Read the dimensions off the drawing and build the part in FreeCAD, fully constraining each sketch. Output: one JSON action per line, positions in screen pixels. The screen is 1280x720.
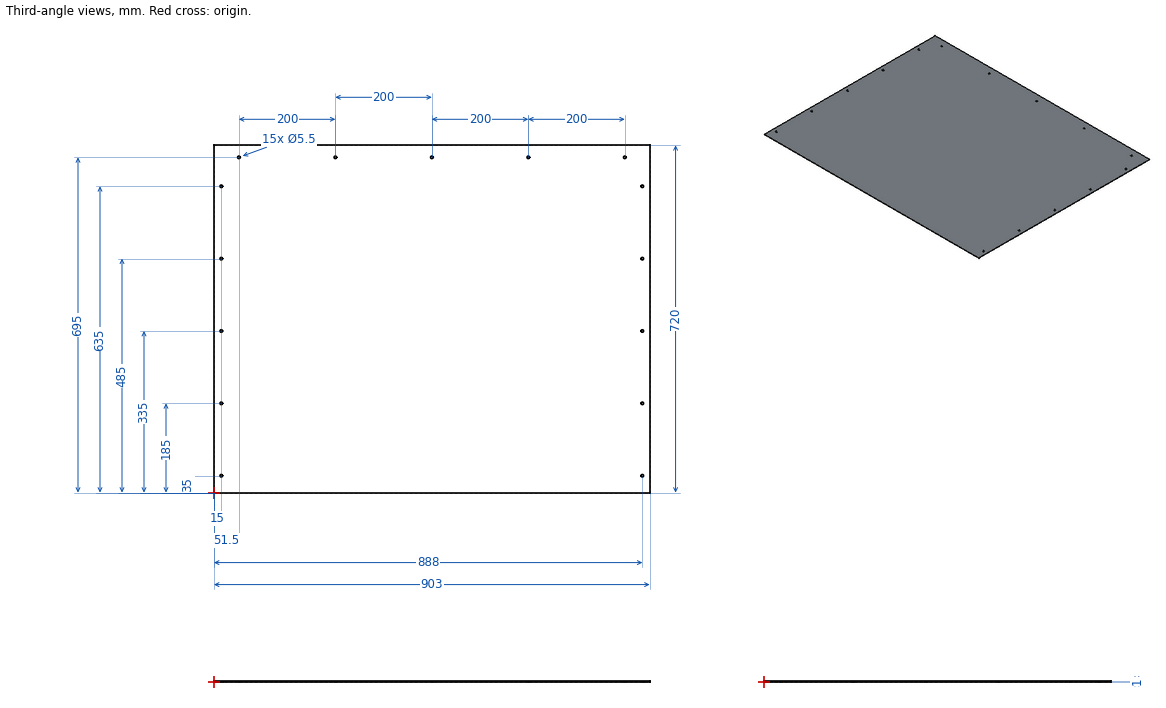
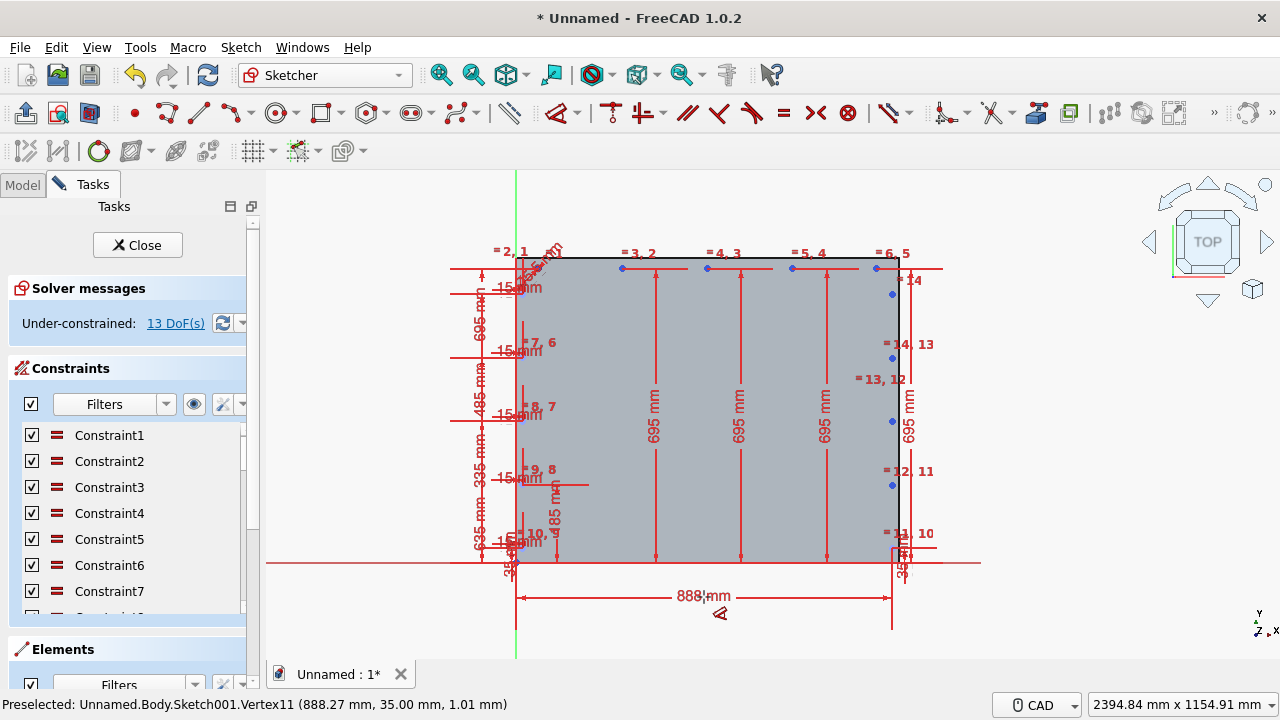
{"action": "left_click", "coordinate": [892, 486]}
{"action": "left_click", "coordinate": [618, 597]}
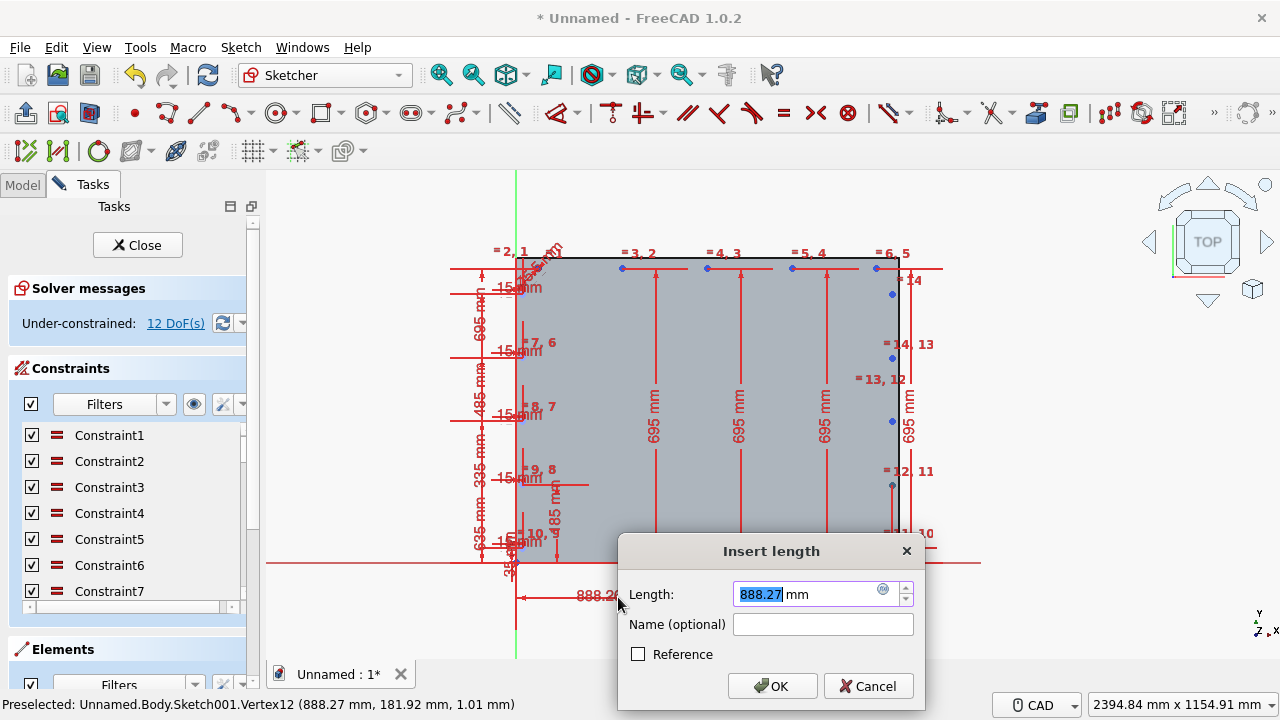
{"action": "type", "text": "888"}
{"action": "key", "text": "Return"}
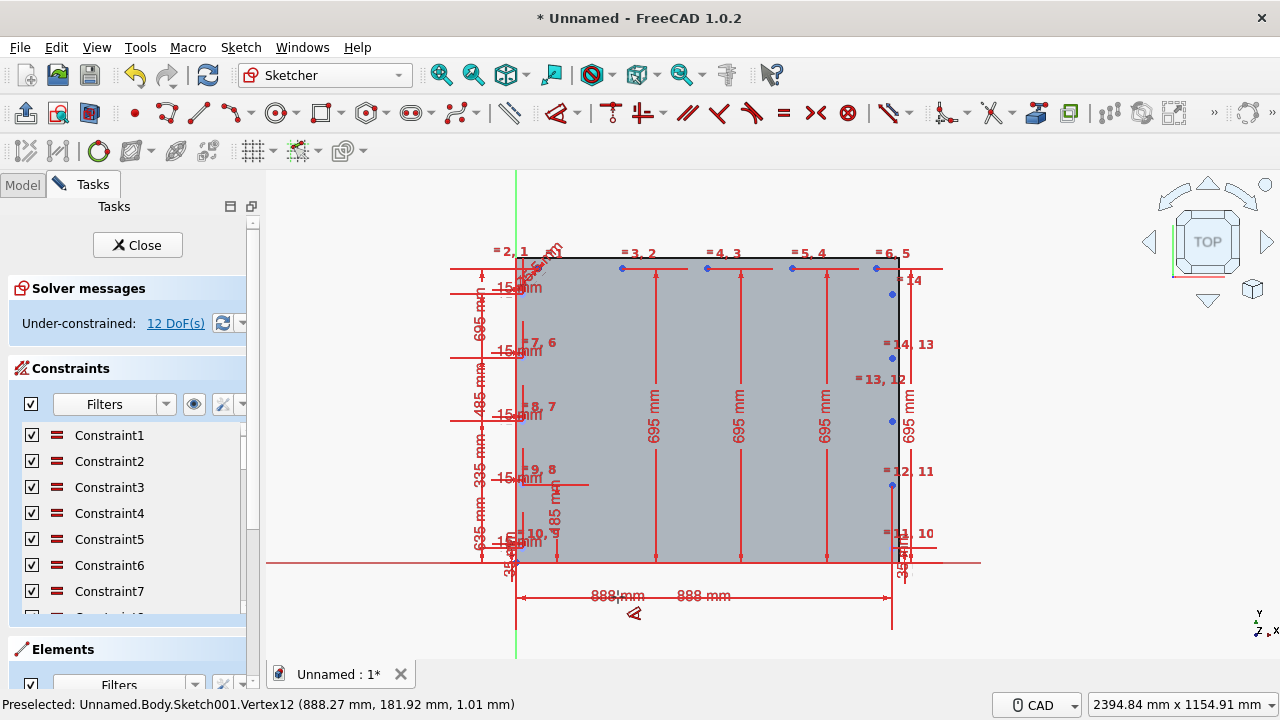
{"action": "left_click", "coordinate": [892, 486]}
{"action": "left_click", "coordinate": [926, 524]}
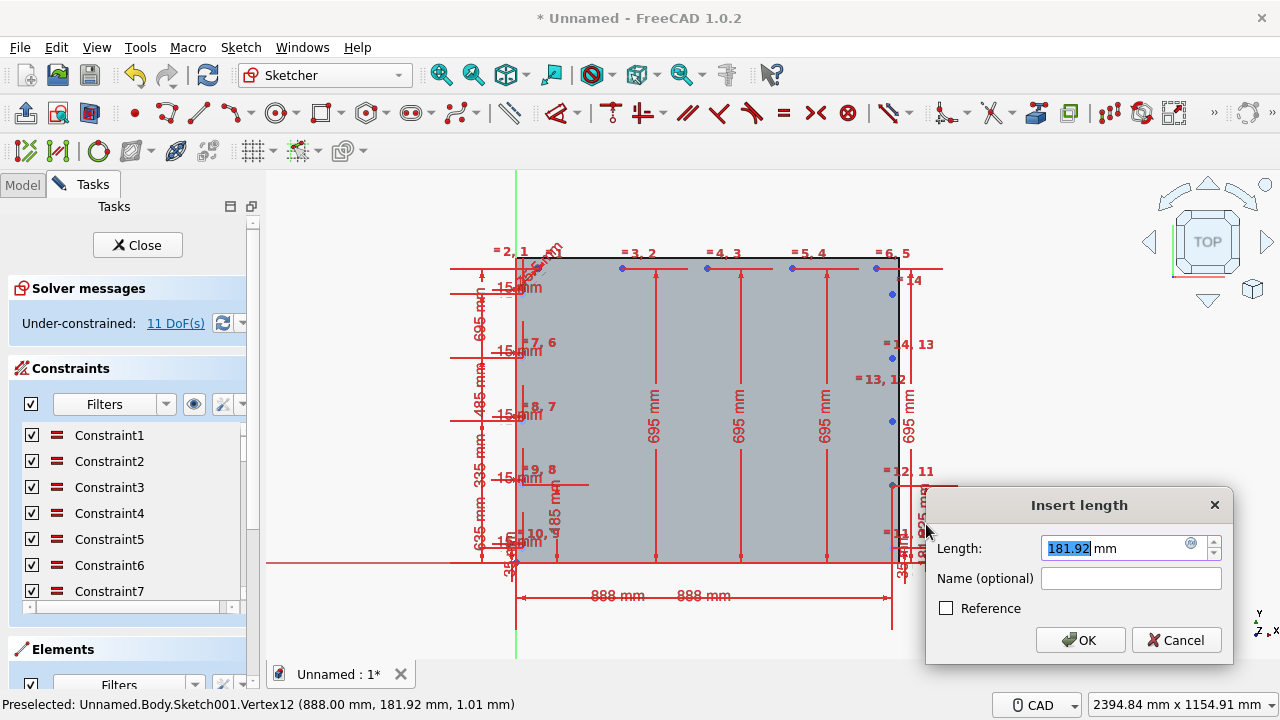
{"action": "type", "text": "185"}
{"action": "key", "text": "Return"}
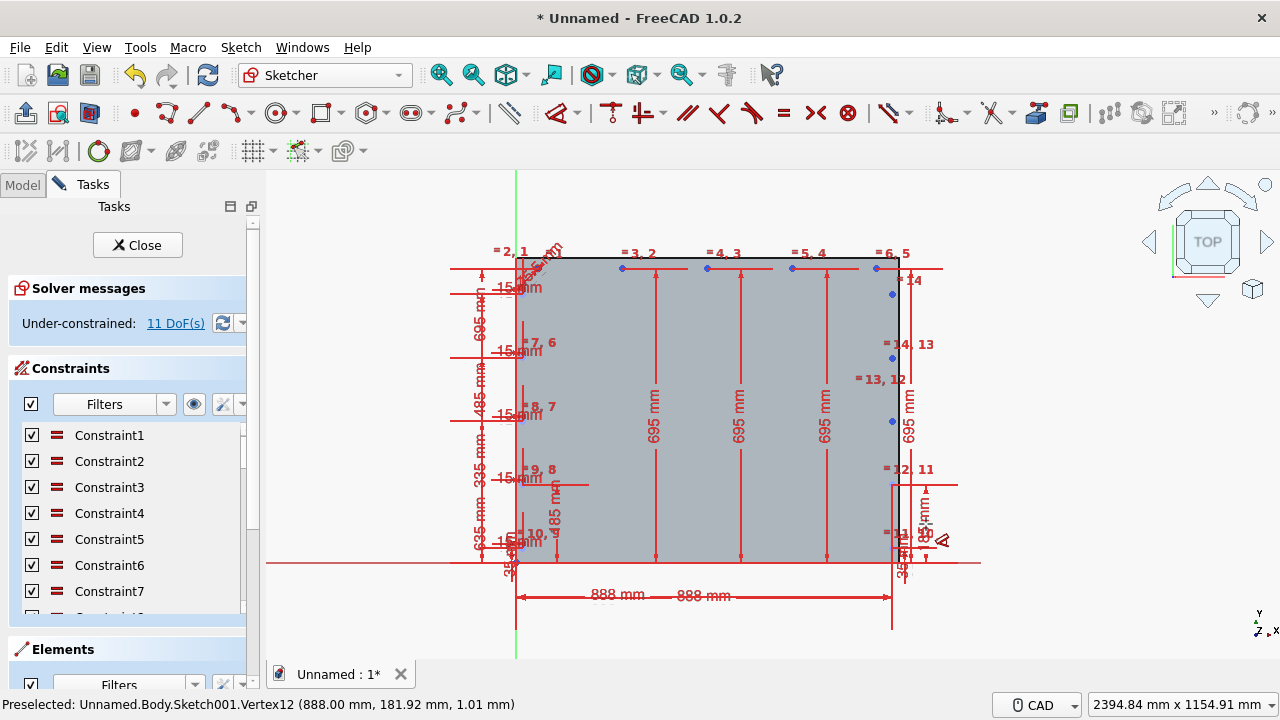
{"action": "left_click", "coordinate": [892, 422]}
{"action": "left_click", "coordinate": [791, 597]}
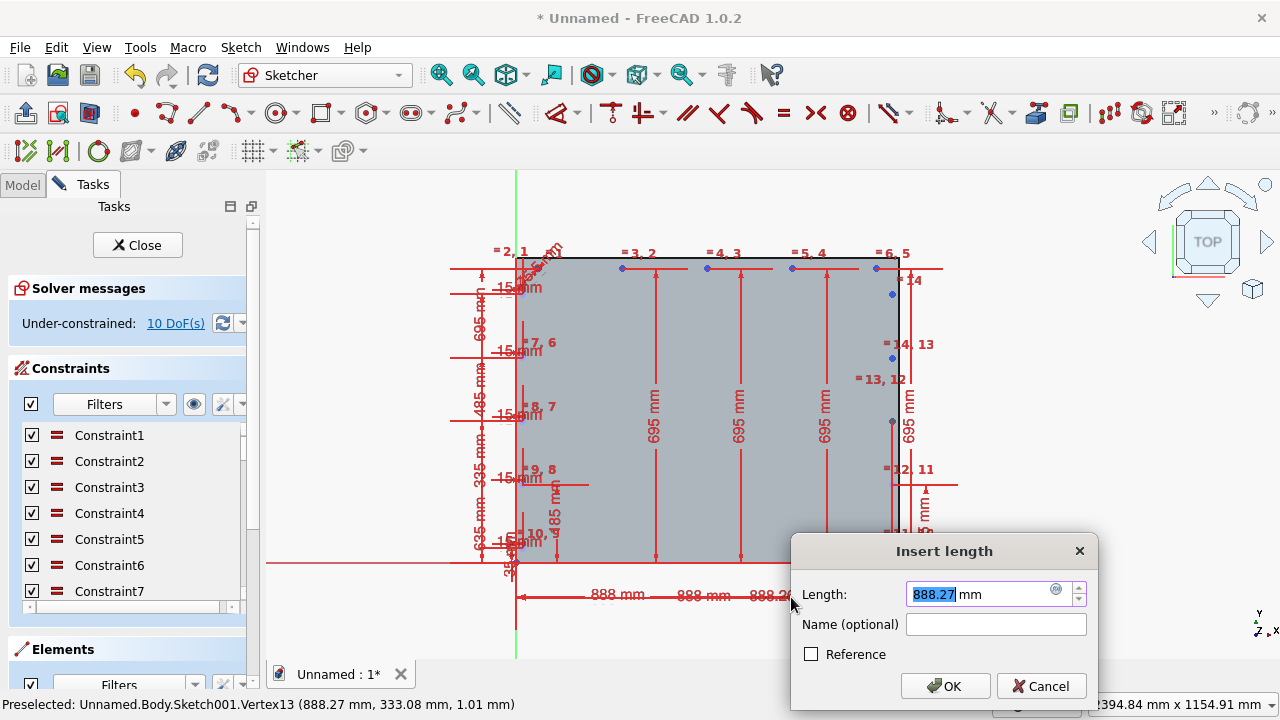
{"action": "type", "text": "888"}
{"action": "key", "text": "Return"}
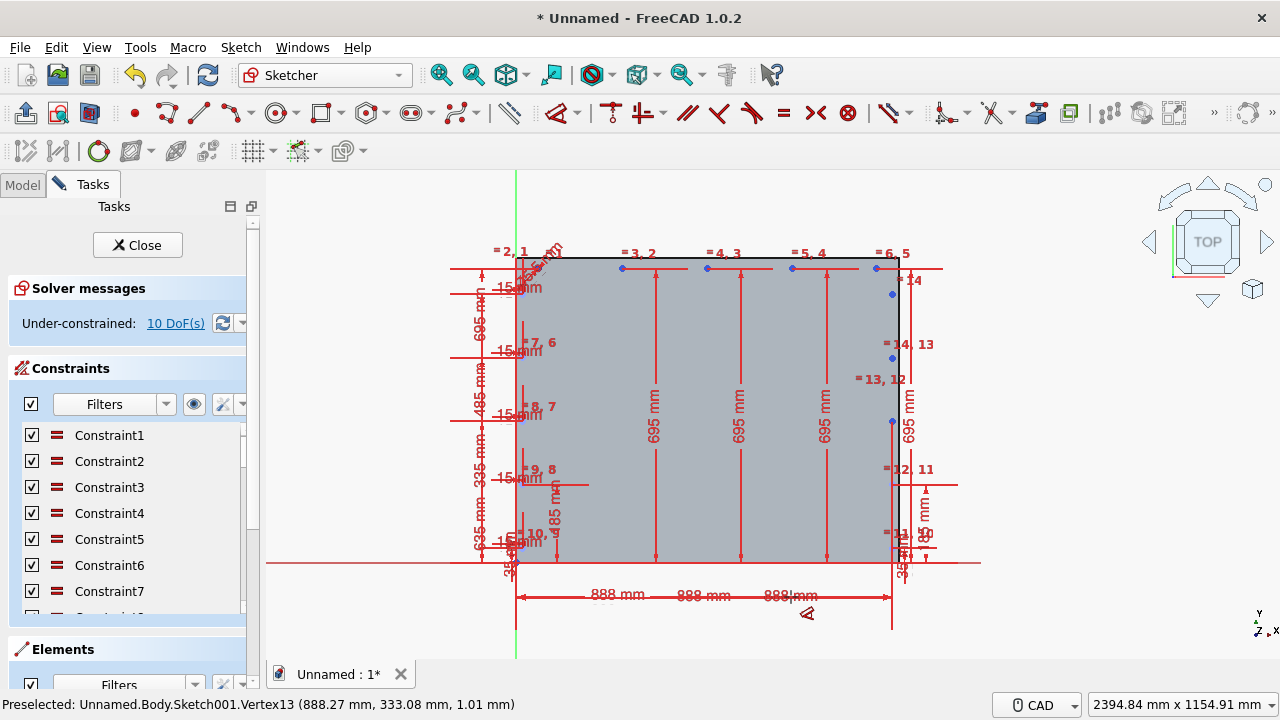
{"action": "left_click", "coordinate": [892, 422]}
{"action": "left_click", "coordinate": [926, 492]}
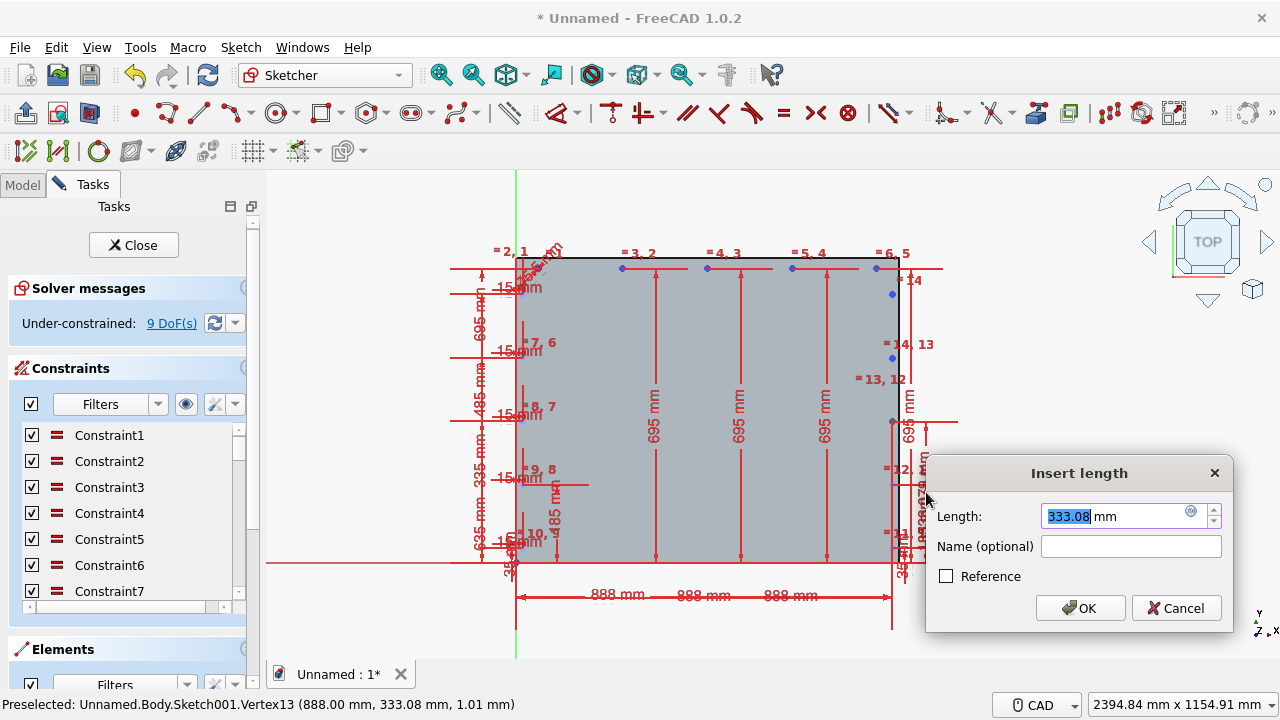
{"action": "type", "text": "335"}
{"action": "key", "text": "Return"}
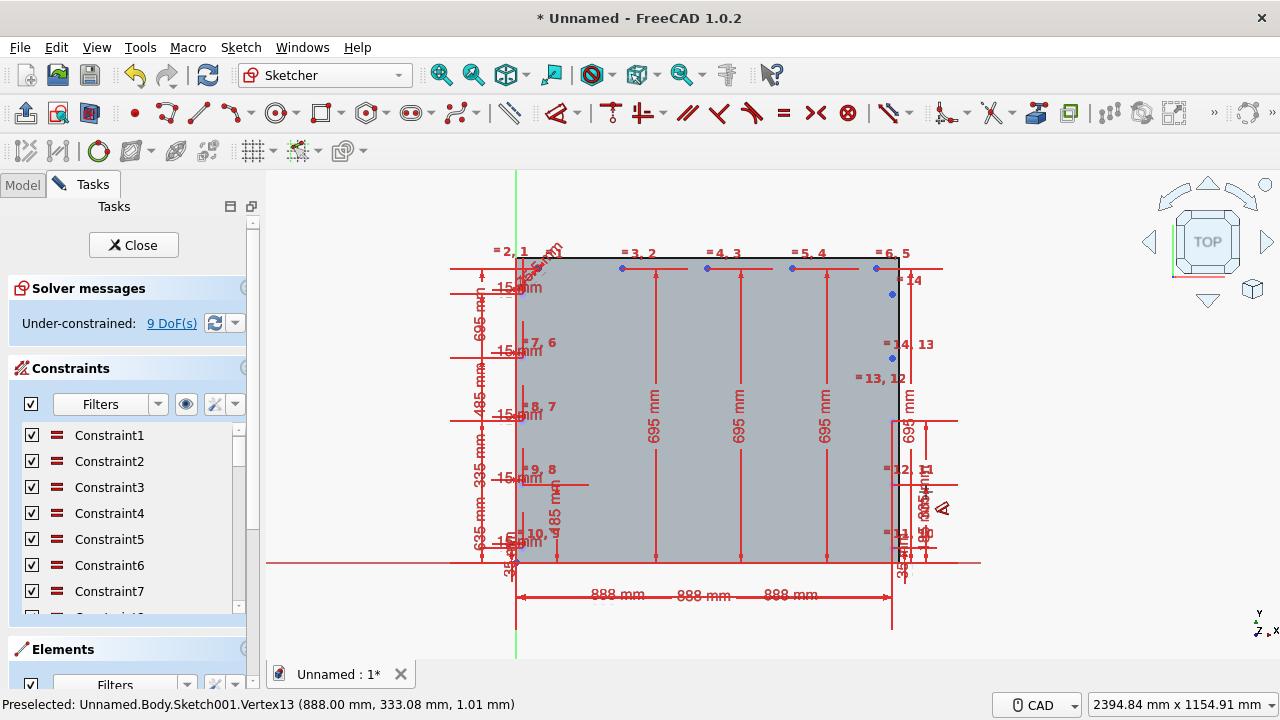
{"action": "left_click", "coordinate": [892, 359]}
{"action": "left_click", "coordinate": [704, 325]}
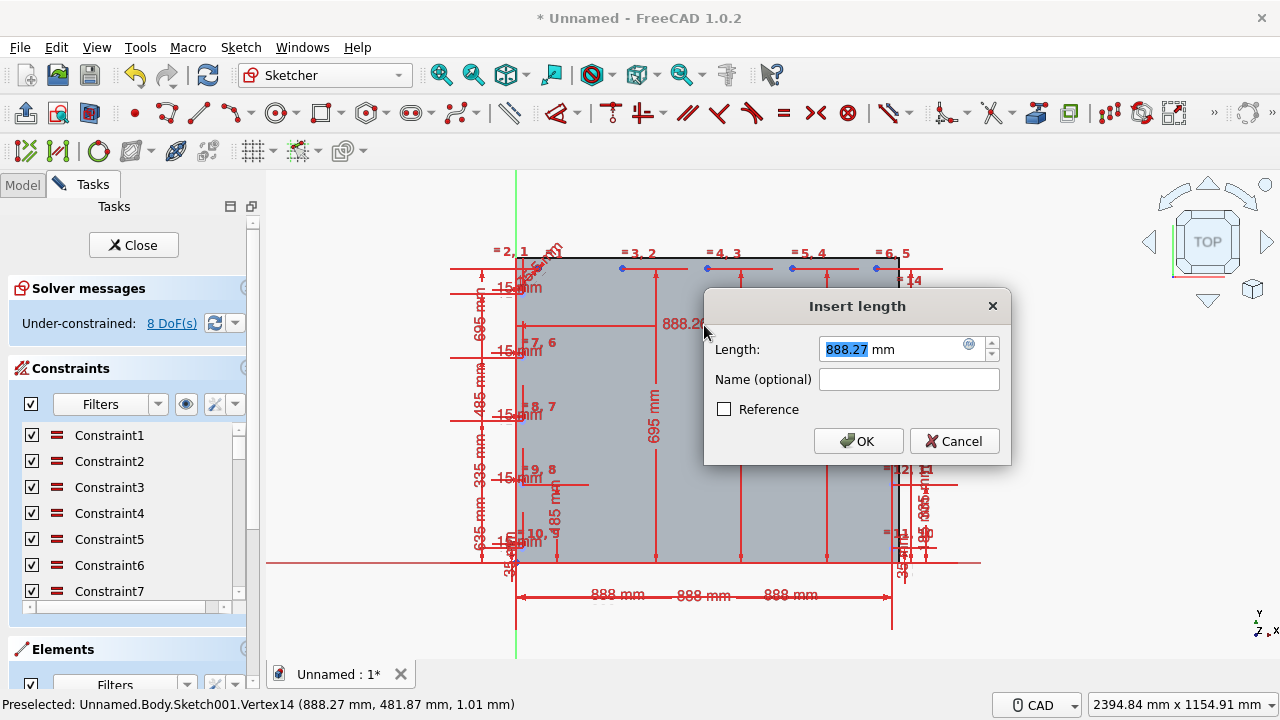
{"action": "type", "text": "888"}
{"action": "key", "text": "Return"}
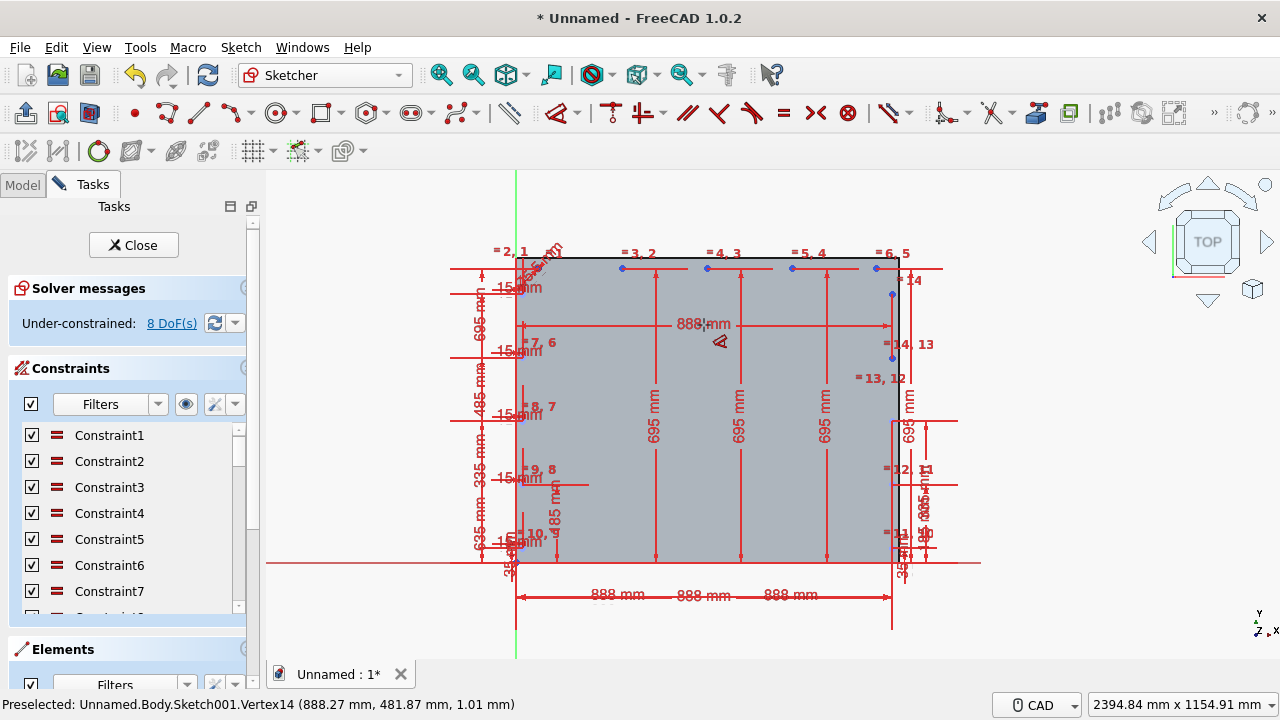
{"action": "left_click", "coordinate": [892, 359]}
{"action": "left_click", "coordinate": [926, 461]}